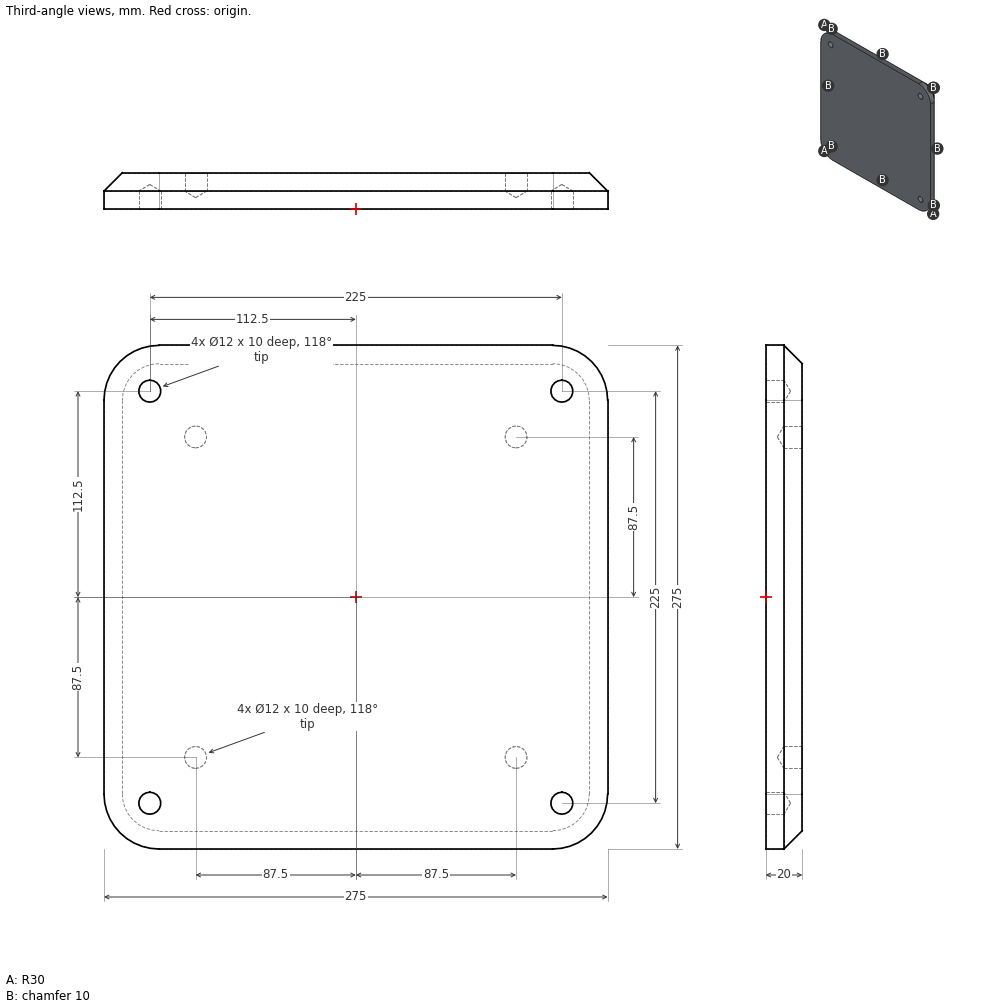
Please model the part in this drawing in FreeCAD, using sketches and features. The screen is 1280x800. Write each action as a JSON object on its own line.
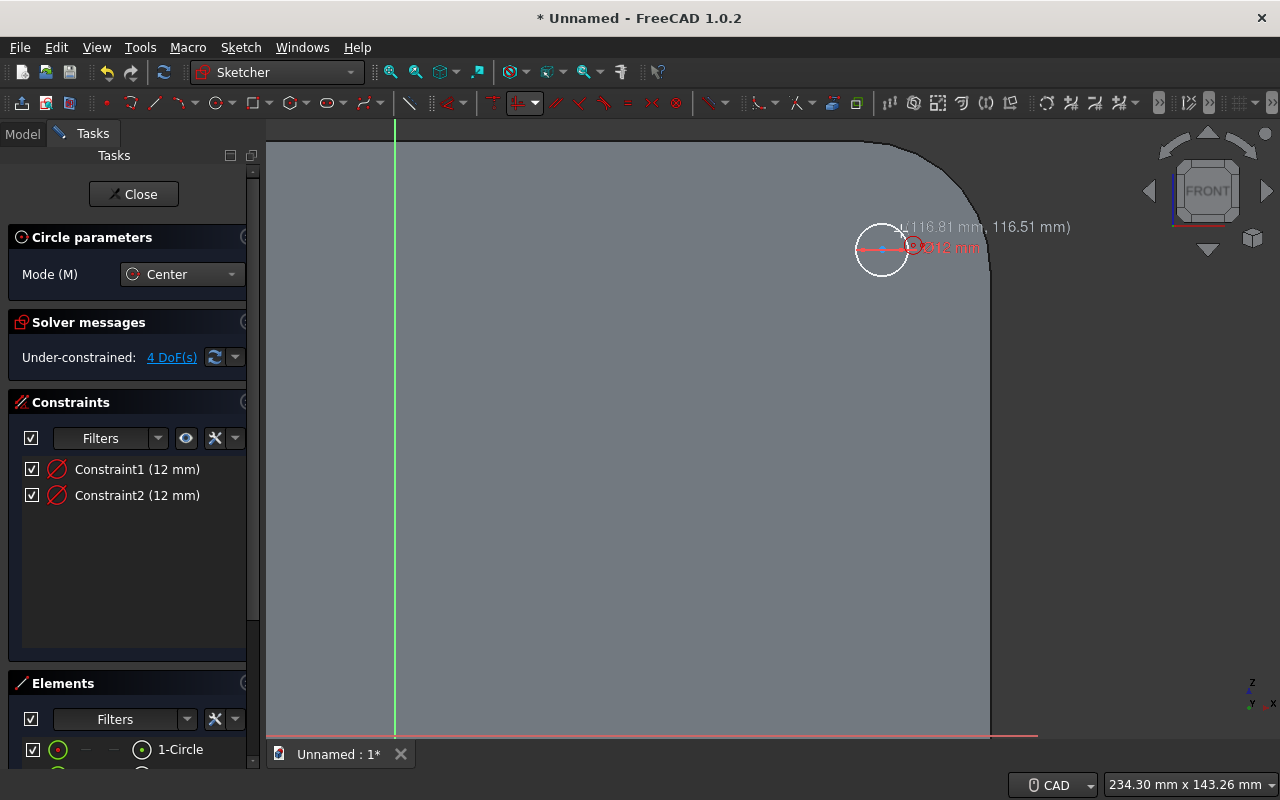
{"action": "scroll", "coordinate": [884, 250], "scroll_direction": "down", "scroll_amount": 5}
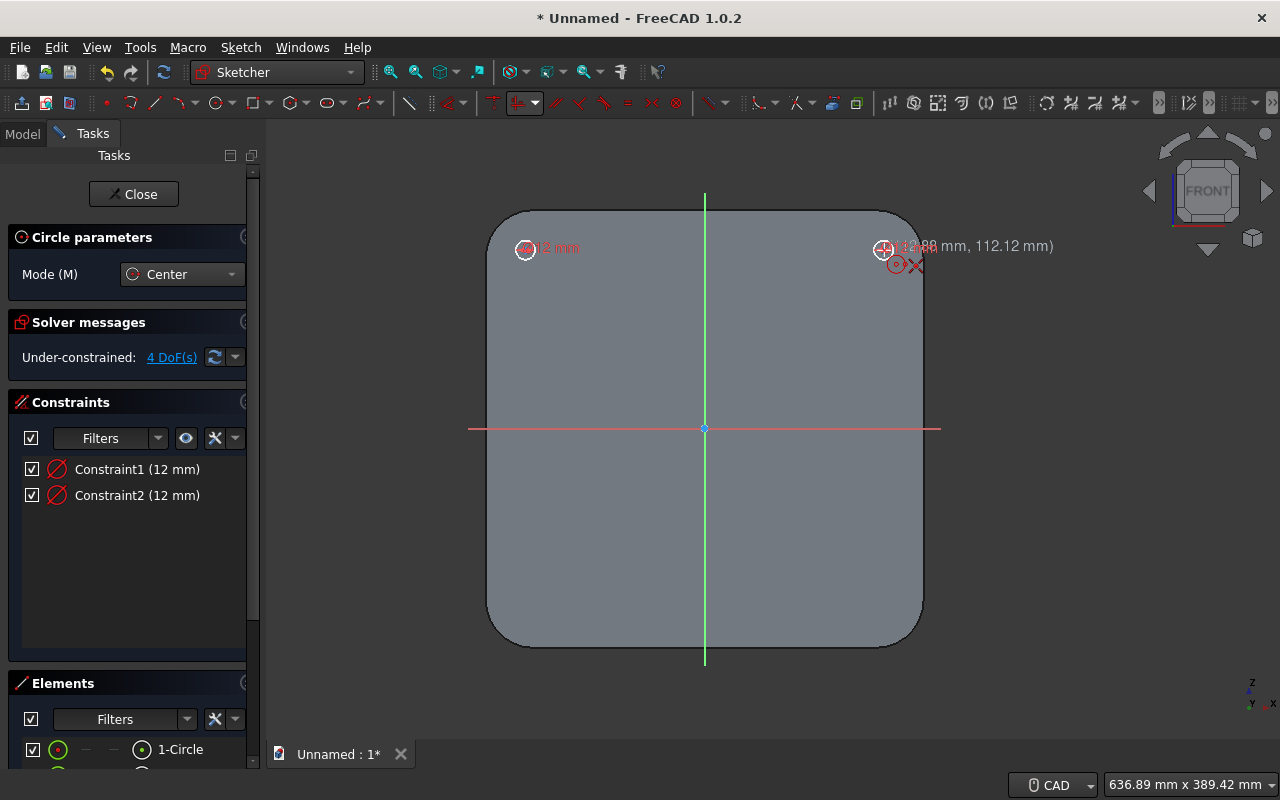
{"action": "scroll", "coordinate": [884, 608], "scroll_direction": "up", "scroll_amount": 5}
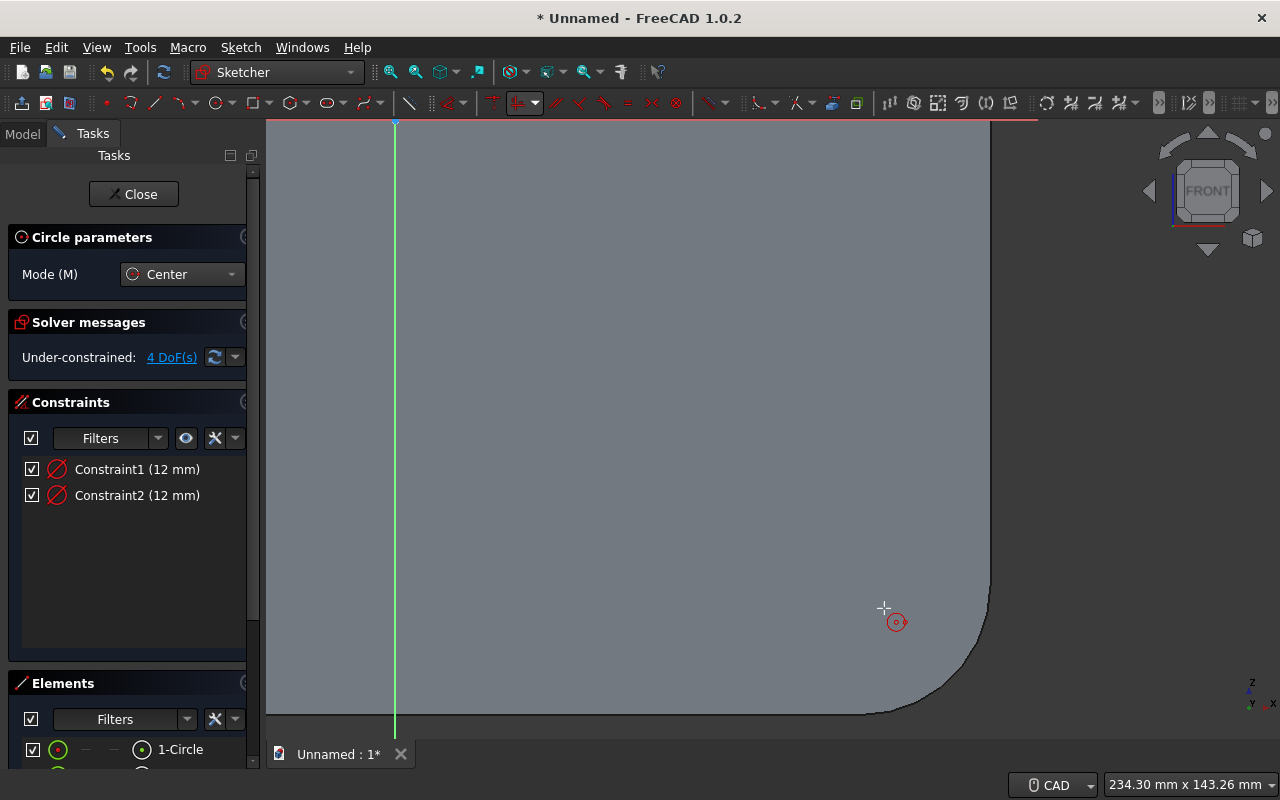
{"action": "left_click", "coordinate": [882, 607]}
{"action": "mouse_move", "coordinate": [901, 589]}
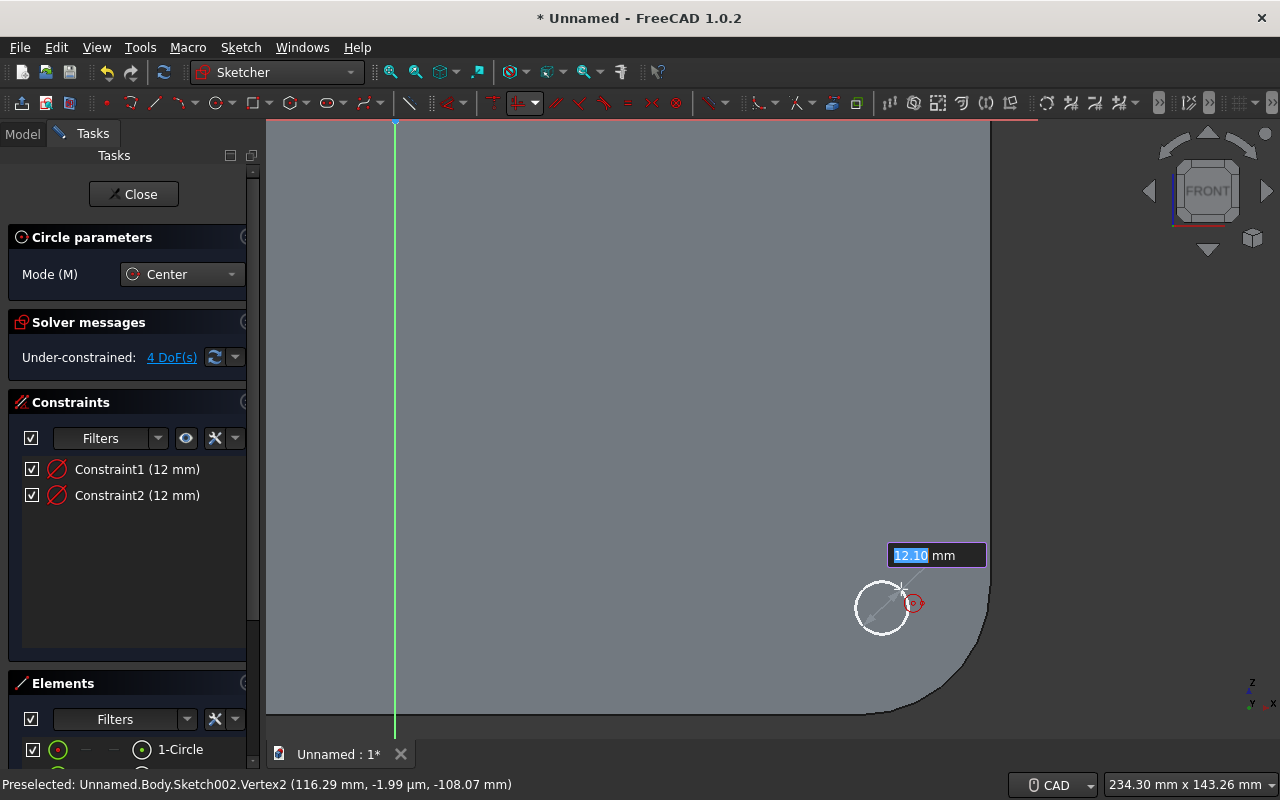
{"action": "type", "text": "12"}
{"action": "key", "text": "Return"}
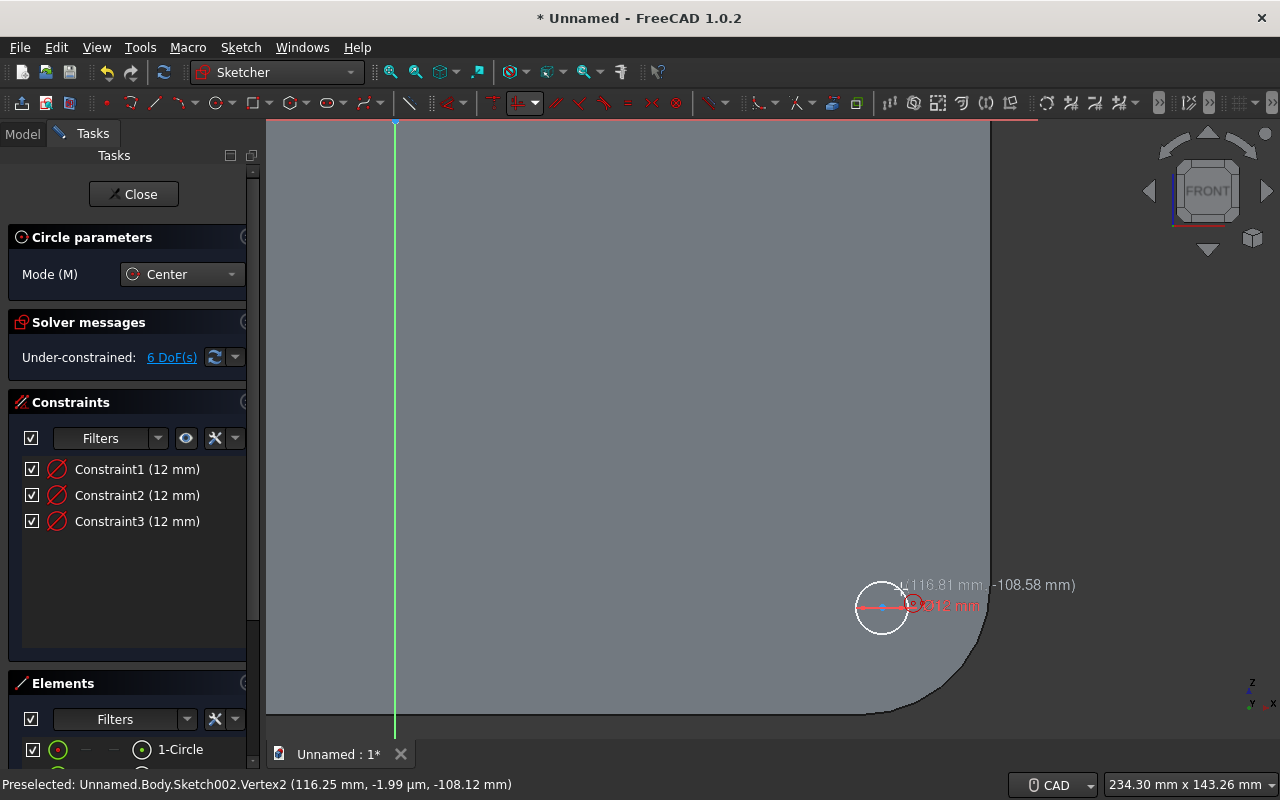
{"action": "scroll", "coordinate": [884, 609], "scroll_direction": "down", "scroll_amount": 5}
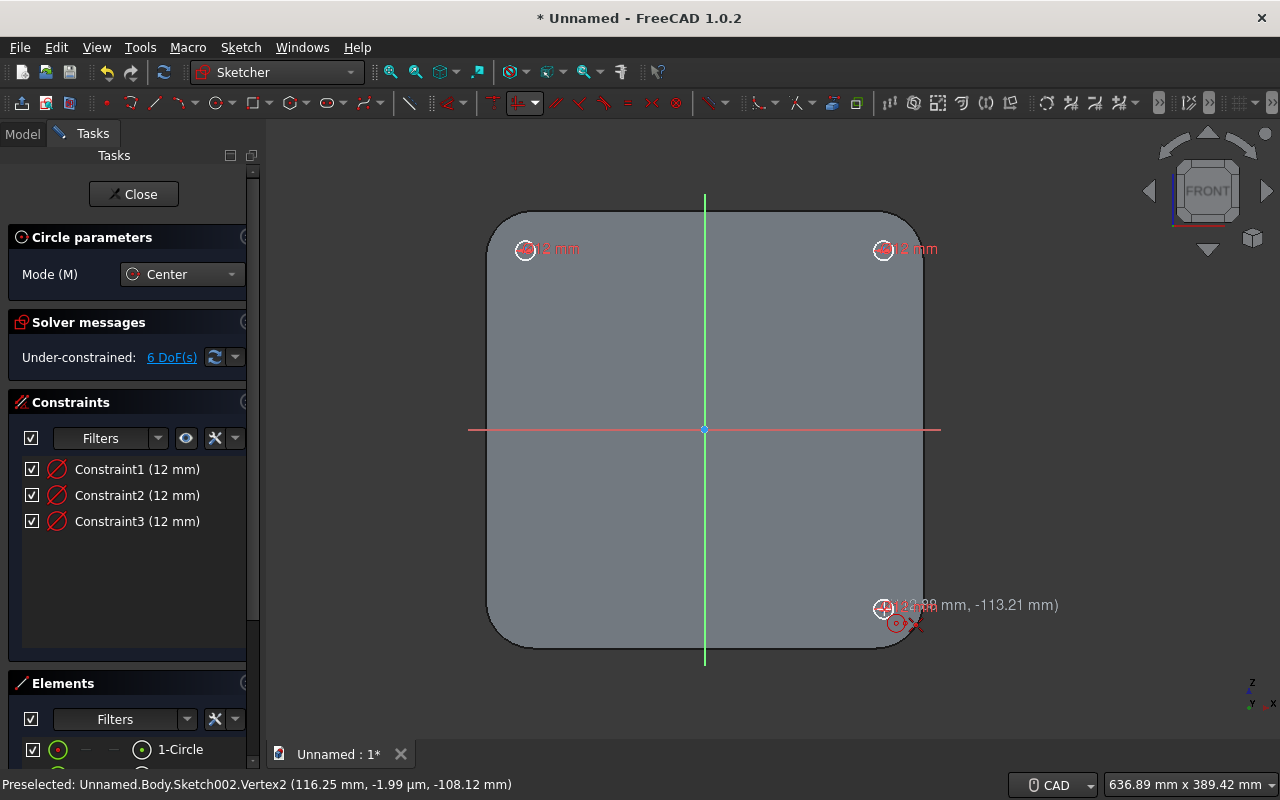
{"action": "scroll", "coordinate": [526, 609], "scroll_direction": "up", "scroll_amount": 5}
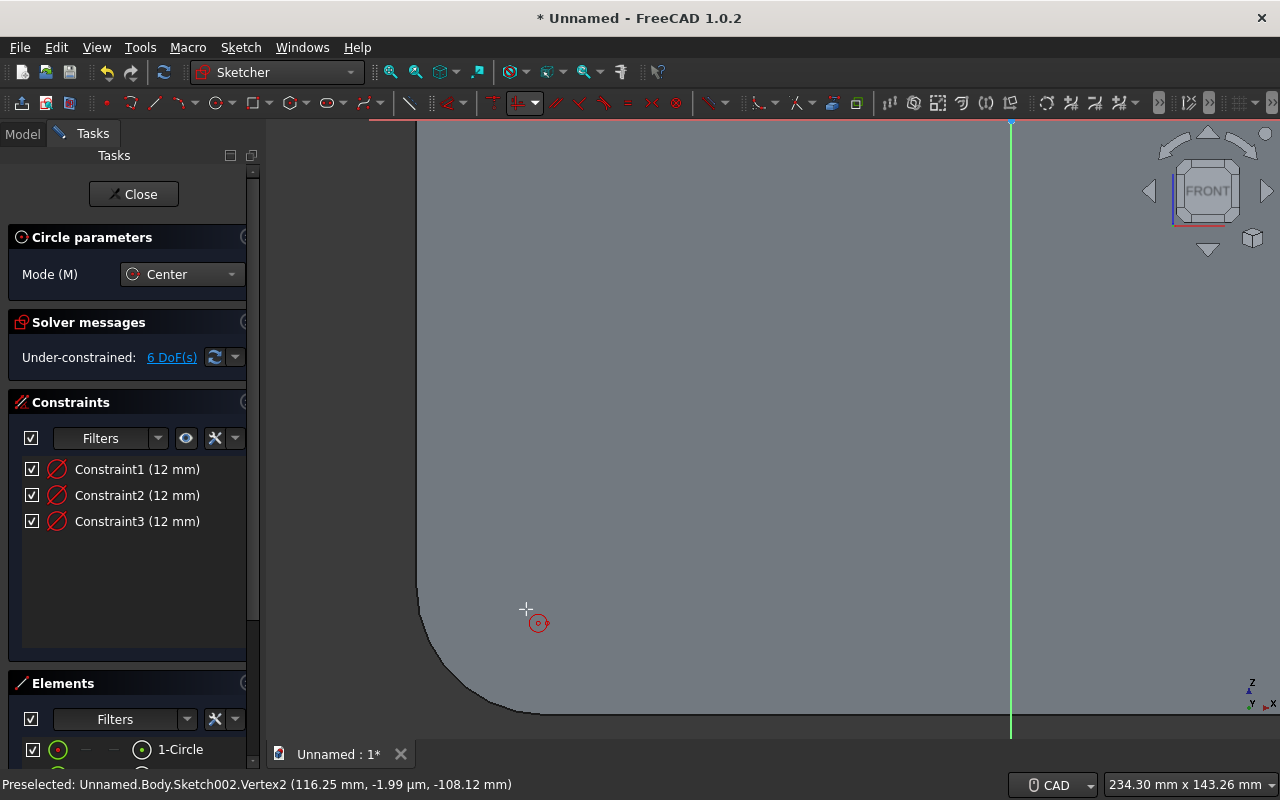
{"action": "left_click", "coordinate": [524, 607]}
{"action": "mouse_move", "coordinate": [543, 589]}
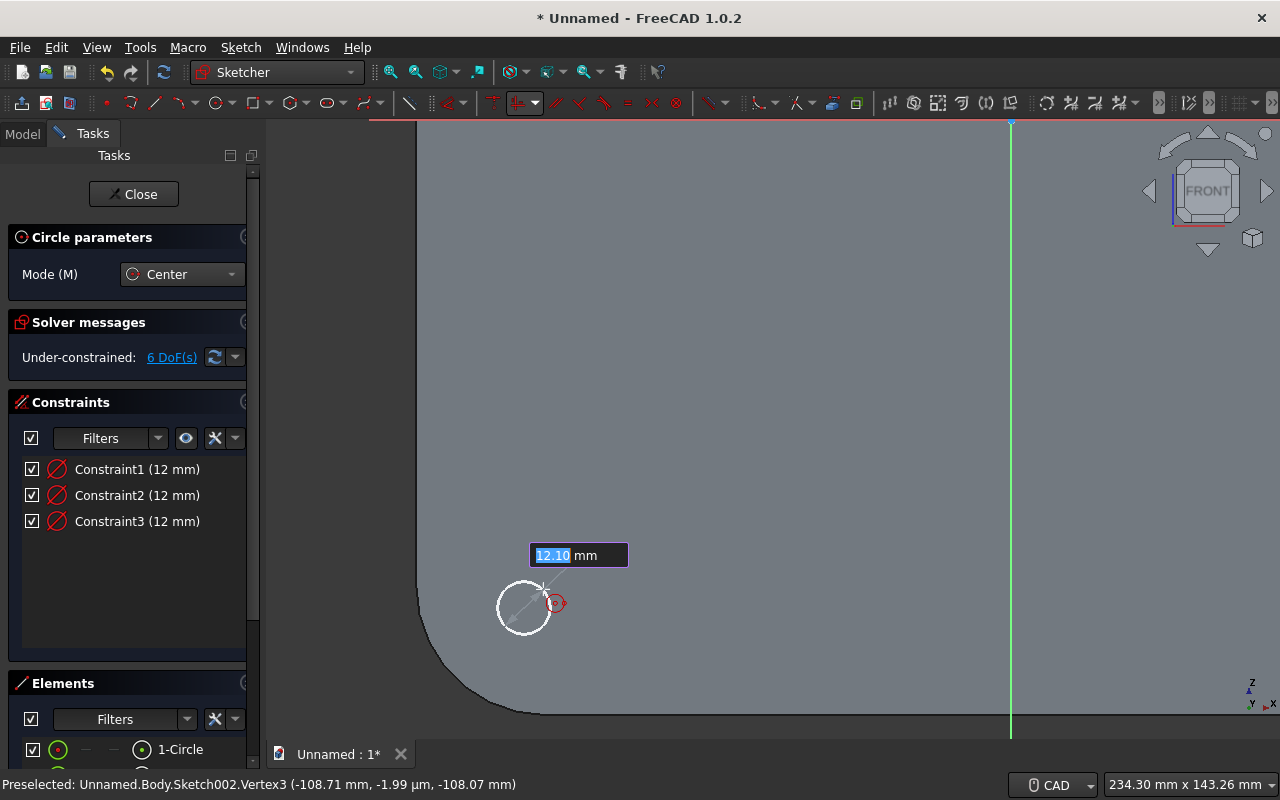
{"action": "type", "text": "12"}
{"action": "key", "text": "Return"}
{"action": "key", "text": "Escape"}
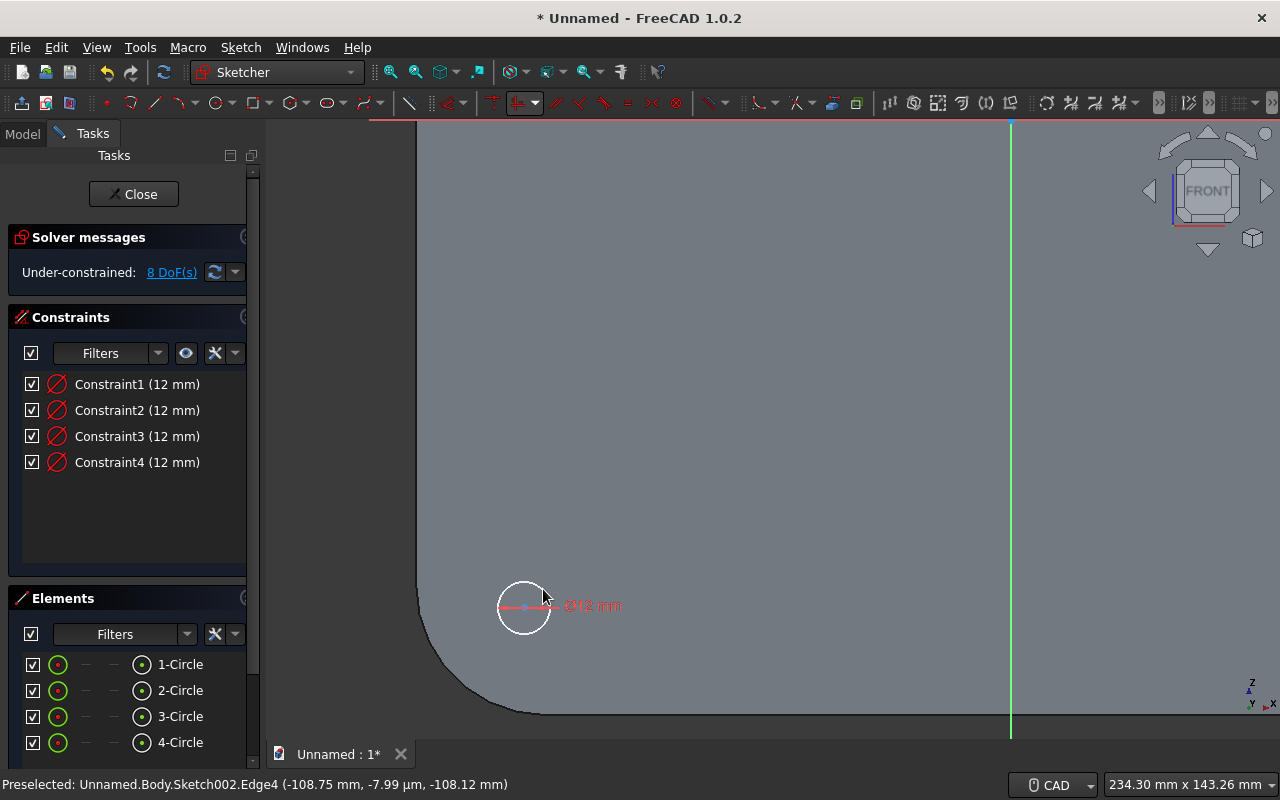
{"action": "scroll", "coordinate": [526, 609], "scroll_direction": "down", "scroll_amount": 5}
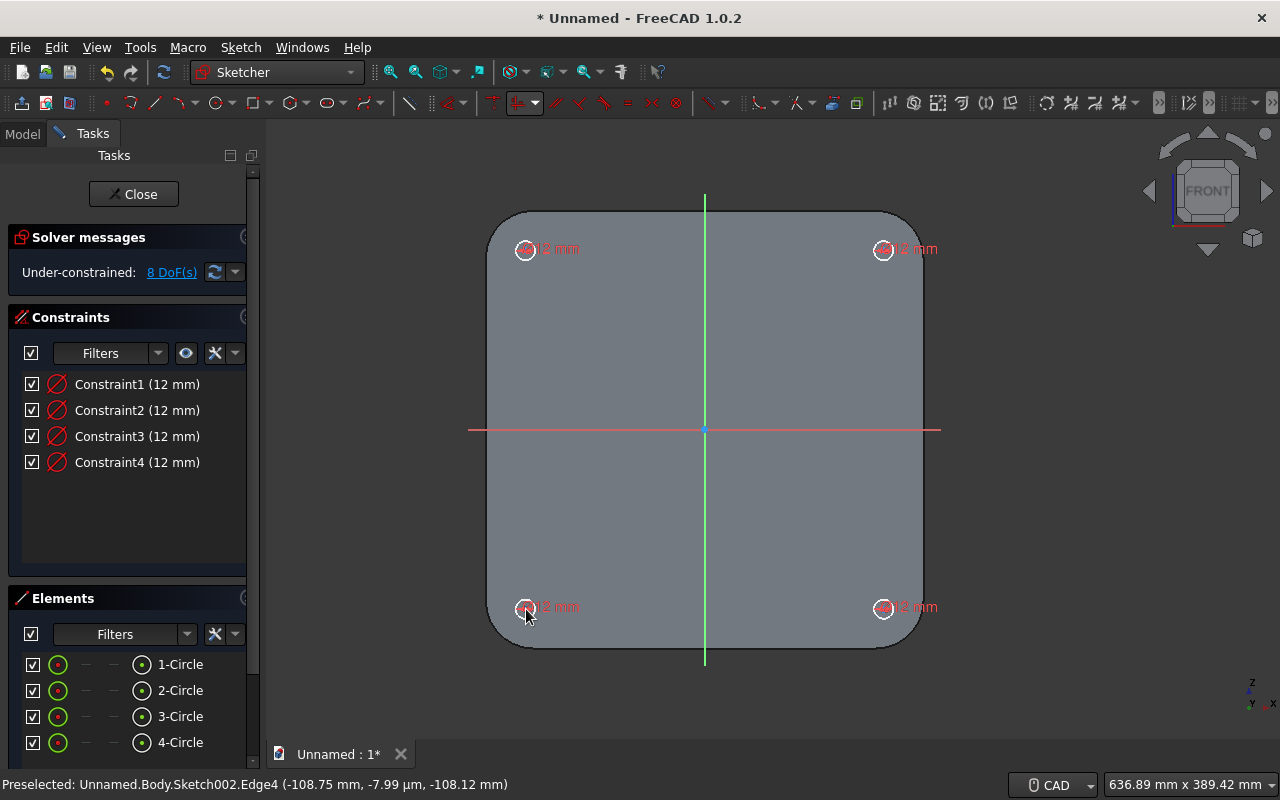
{"action": "left_click", "coordinate": [526, 251]}